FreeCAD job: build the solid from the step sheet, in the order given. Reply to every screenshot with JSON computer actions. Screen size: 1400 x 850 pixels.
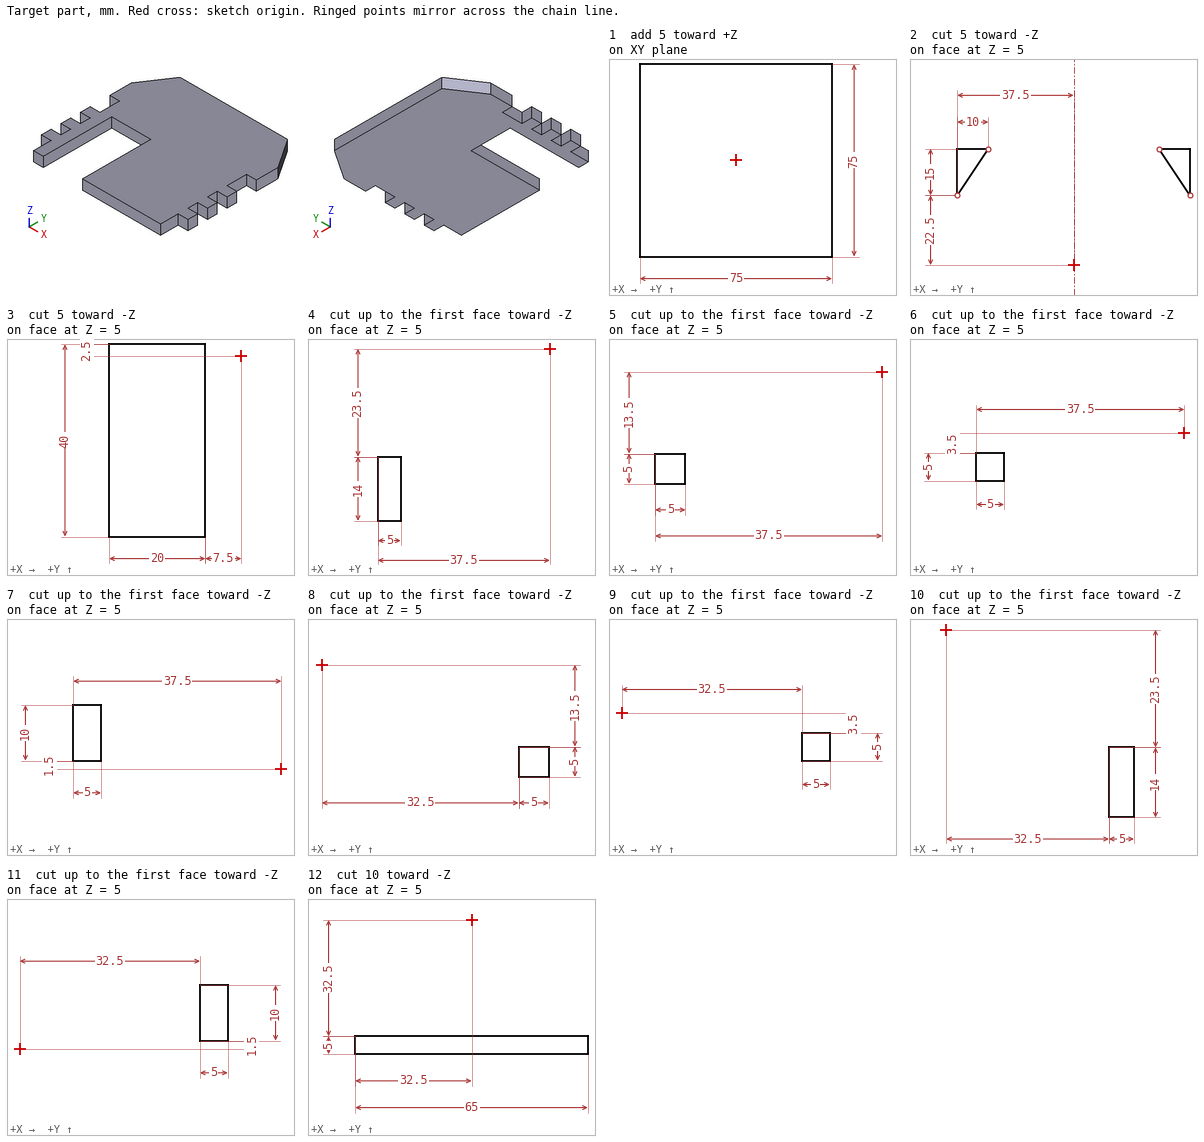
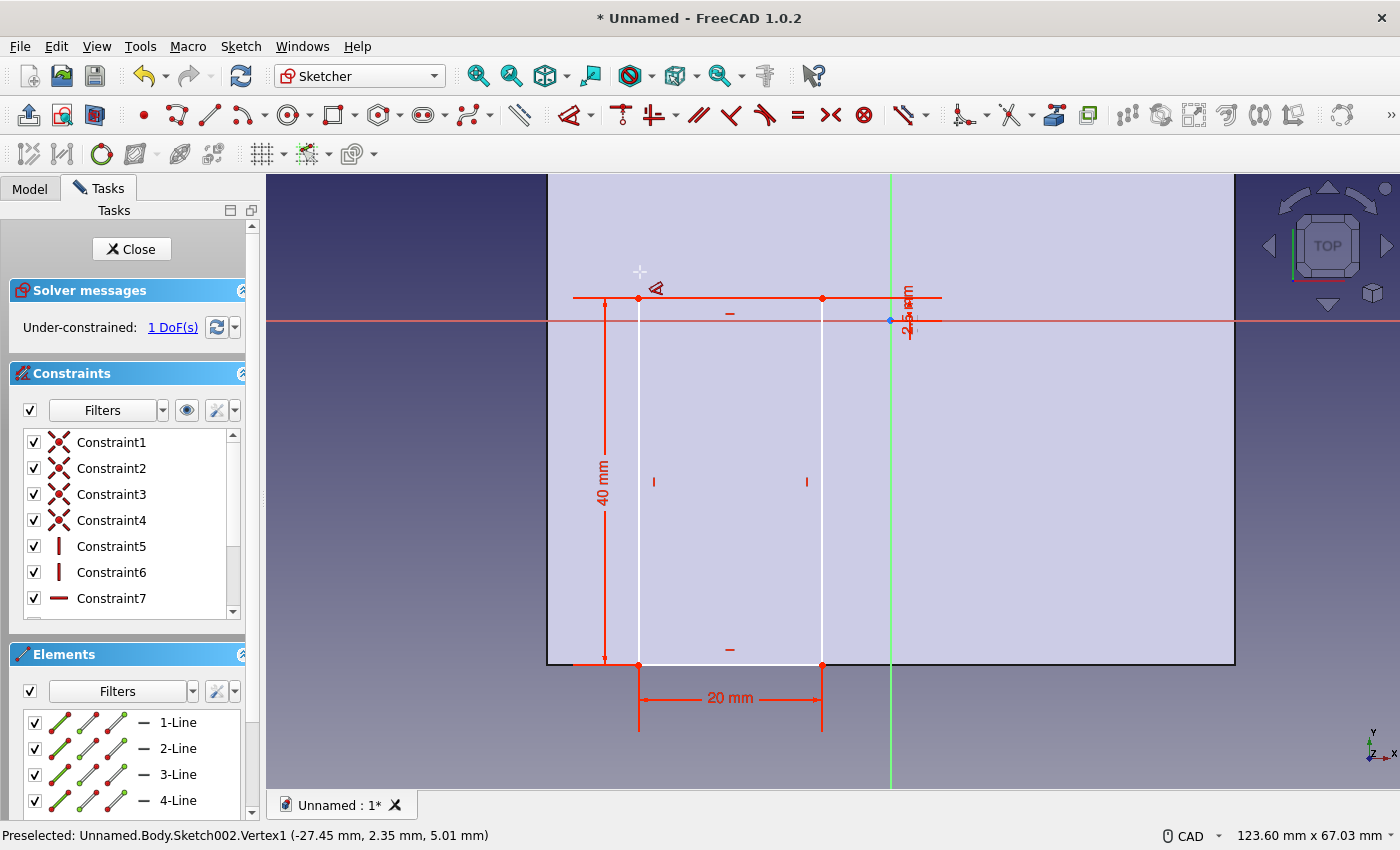
{"action": "left_click", "coordinate": [822, 665]}
{"action": "left_click", "coordinate": [857, 699]}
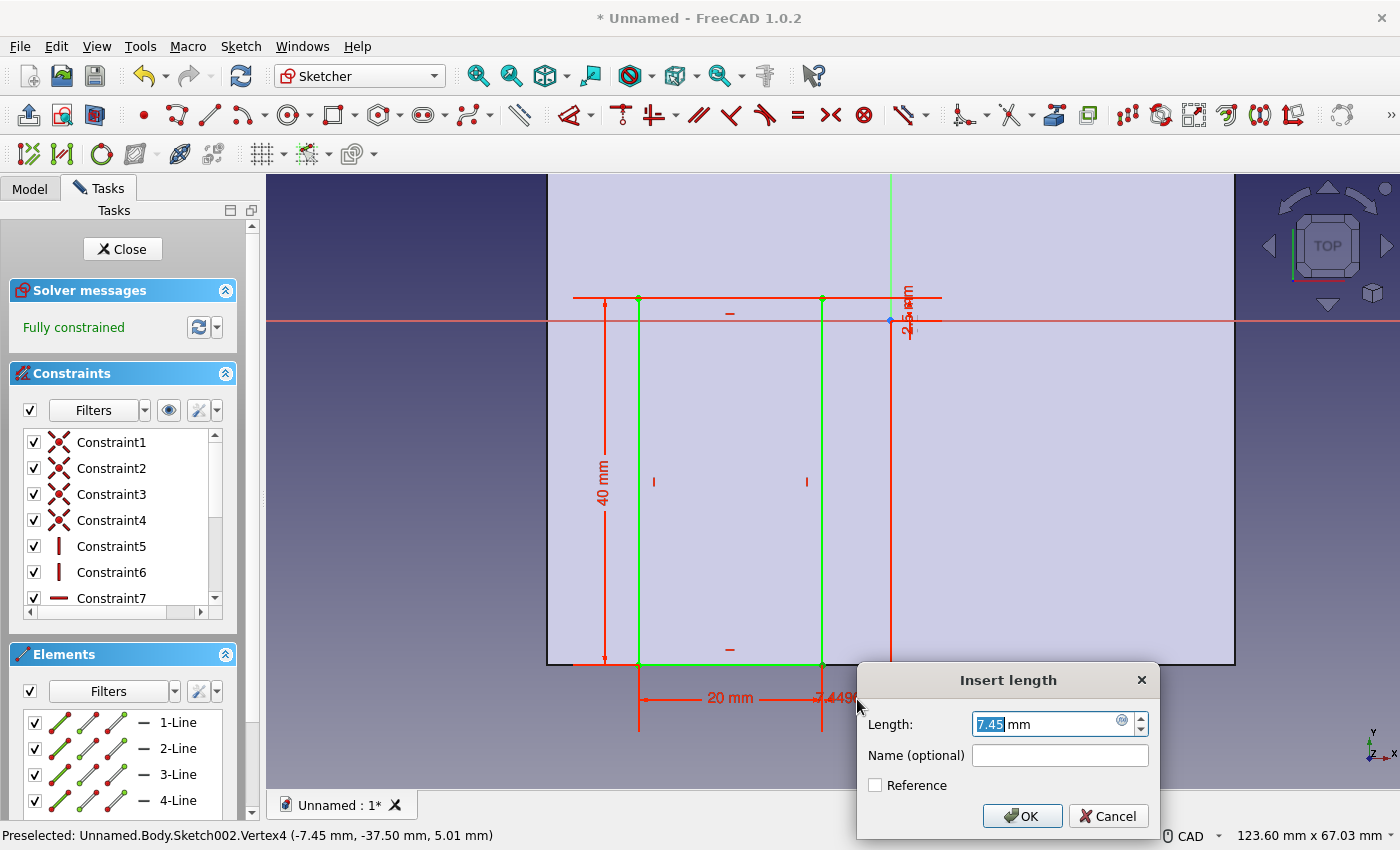
{"action": "type", "text": "7.5"}
{"action": "key", "text": "Return"}
{"action": "key", "text": "Escape"}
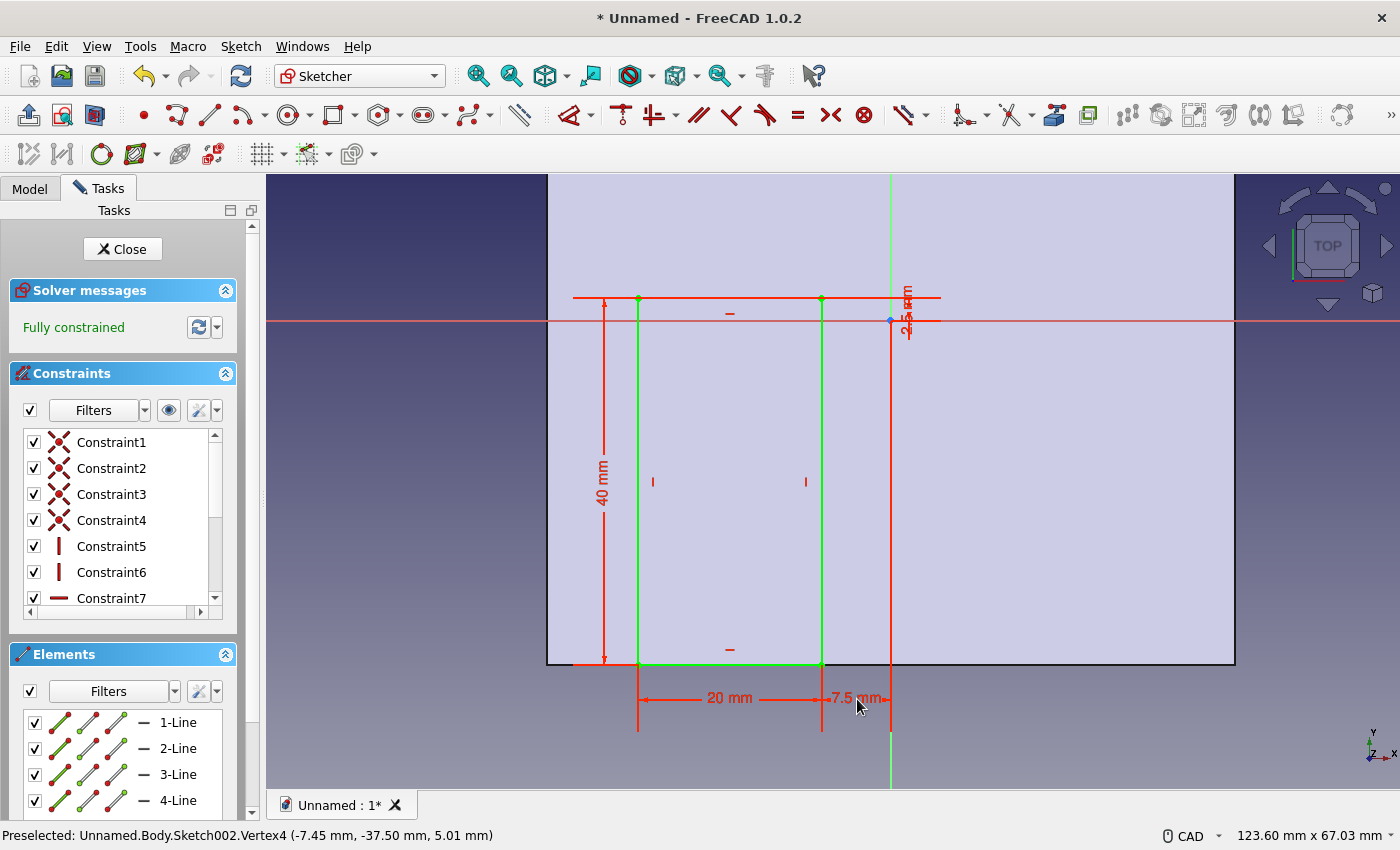
{"action": "left_click", "coordinate": [123, 249]}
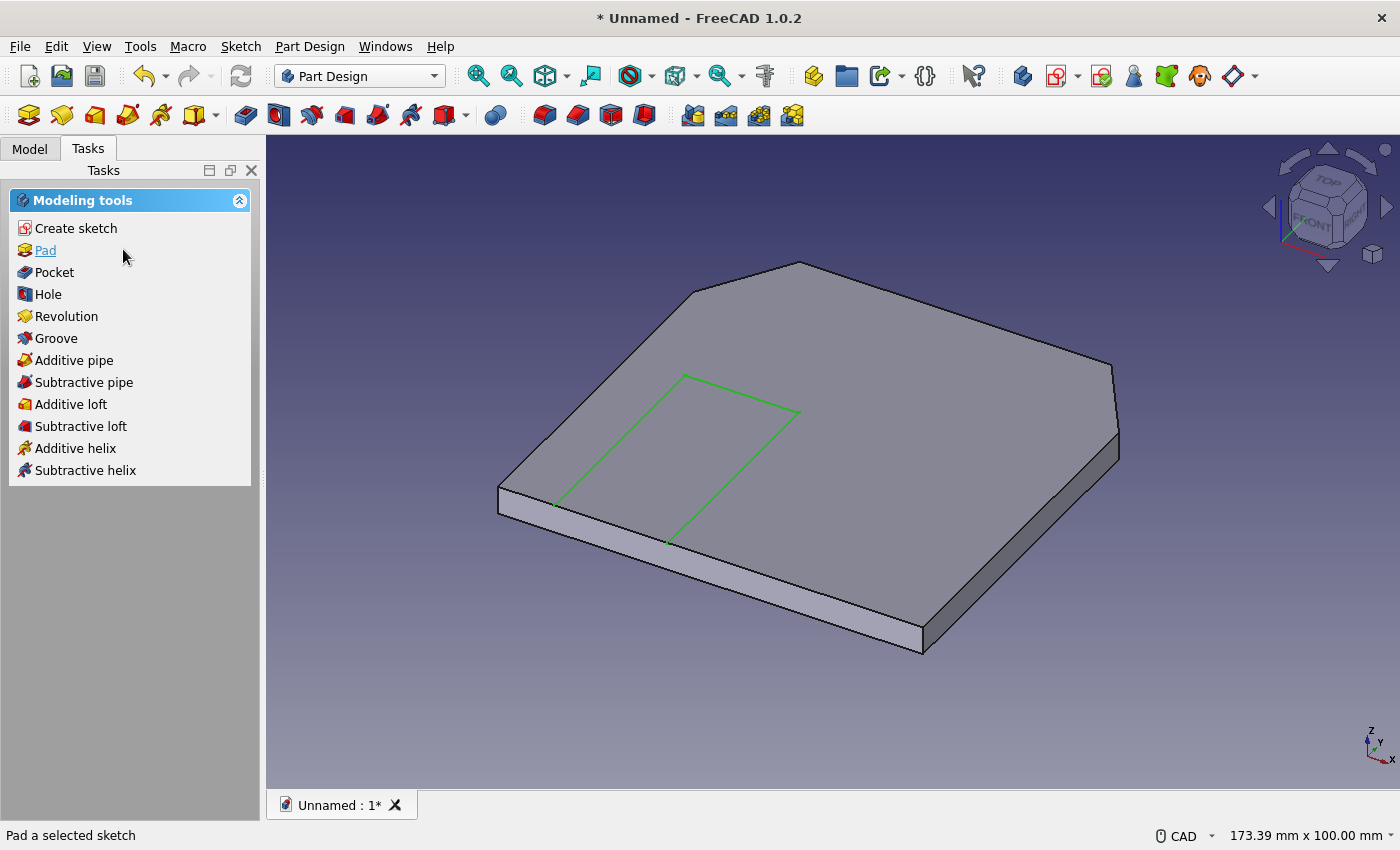
{"action": "left_click", "coordinate": [246, 116]}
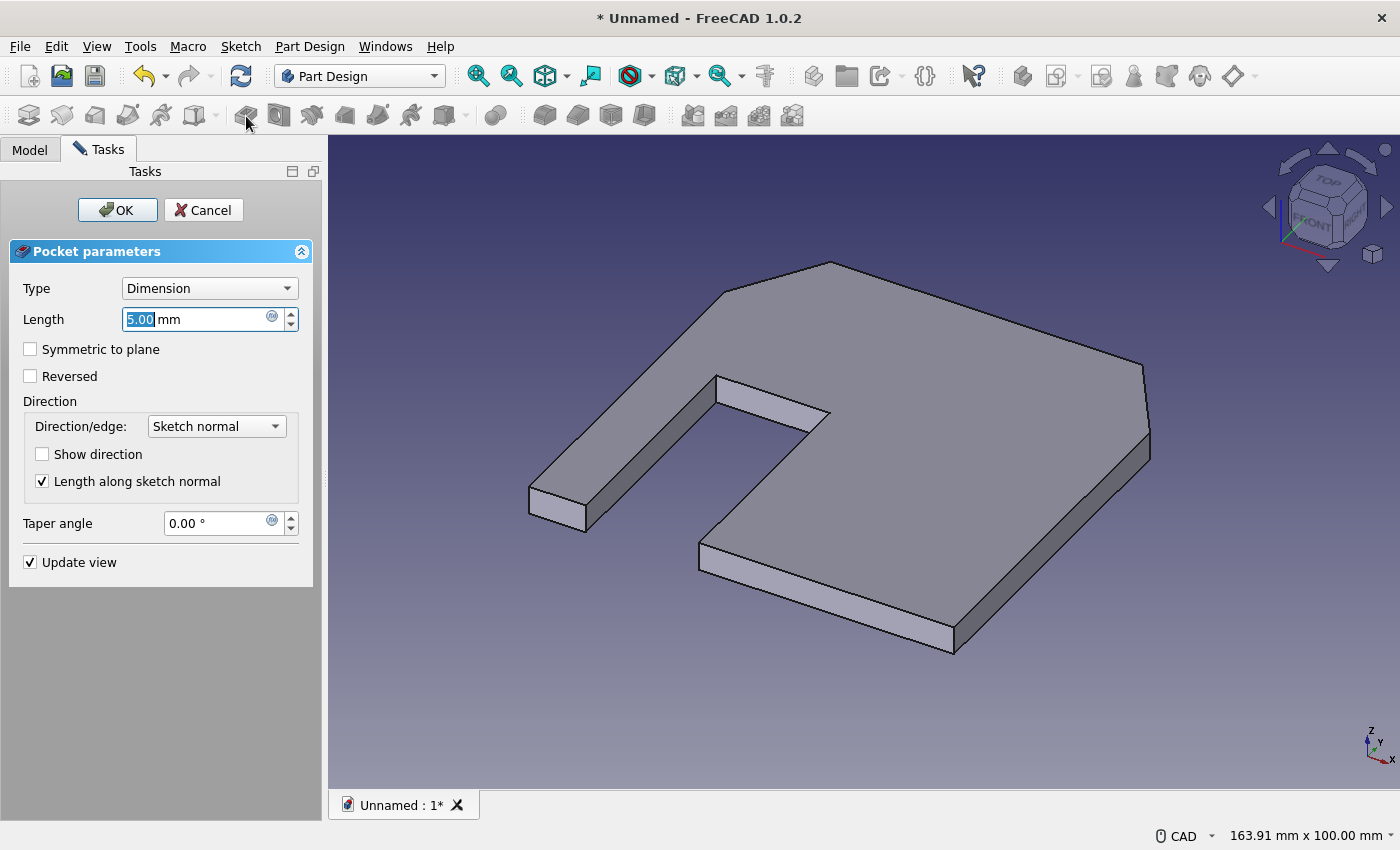
{"action": "type", "text": "5"}
{"action": "key", "text": "Tab"}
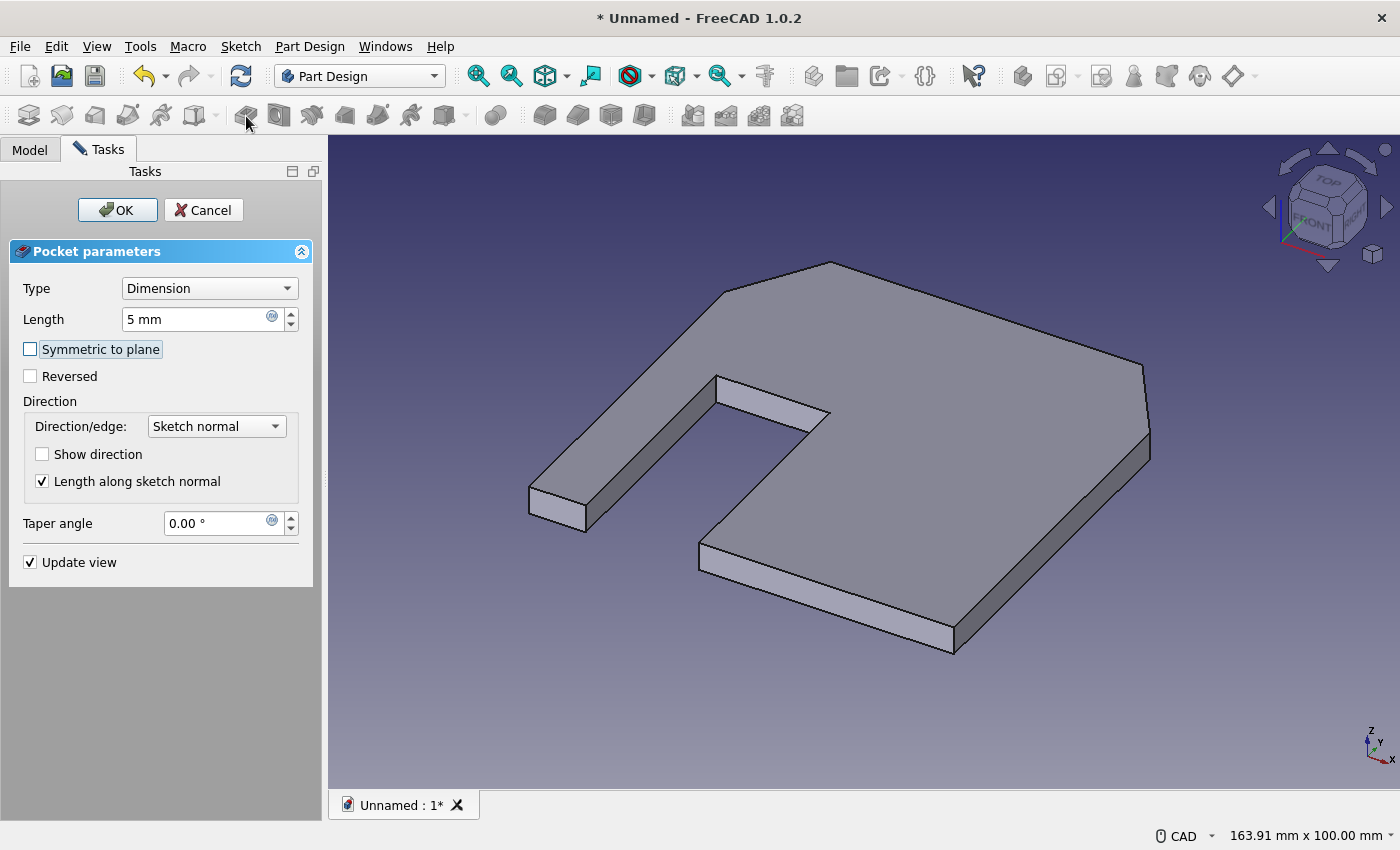
{"action": "left_click", "coordinate": [118, 210]}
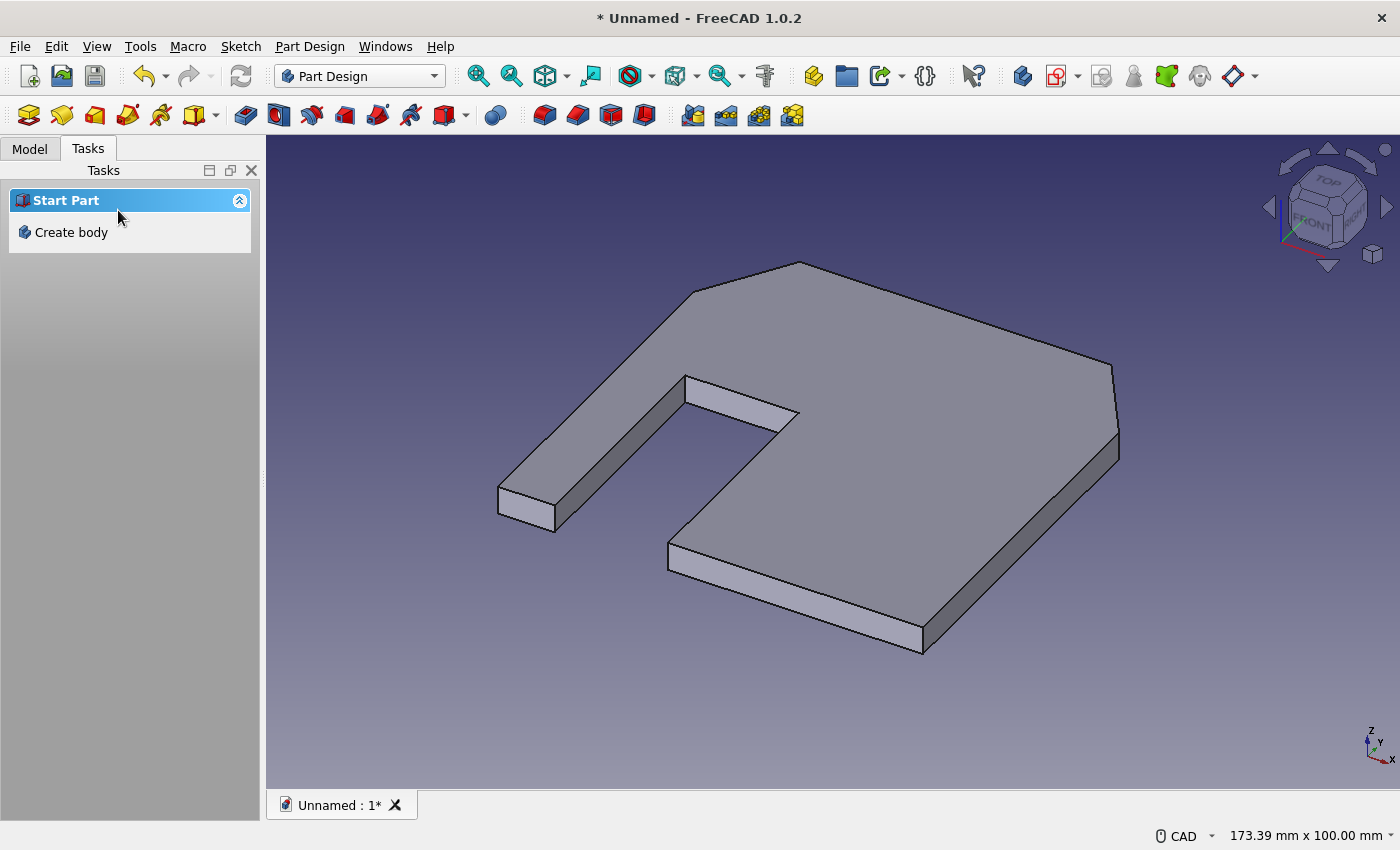
{"action": "left_click", "coordinate": [929, 420]}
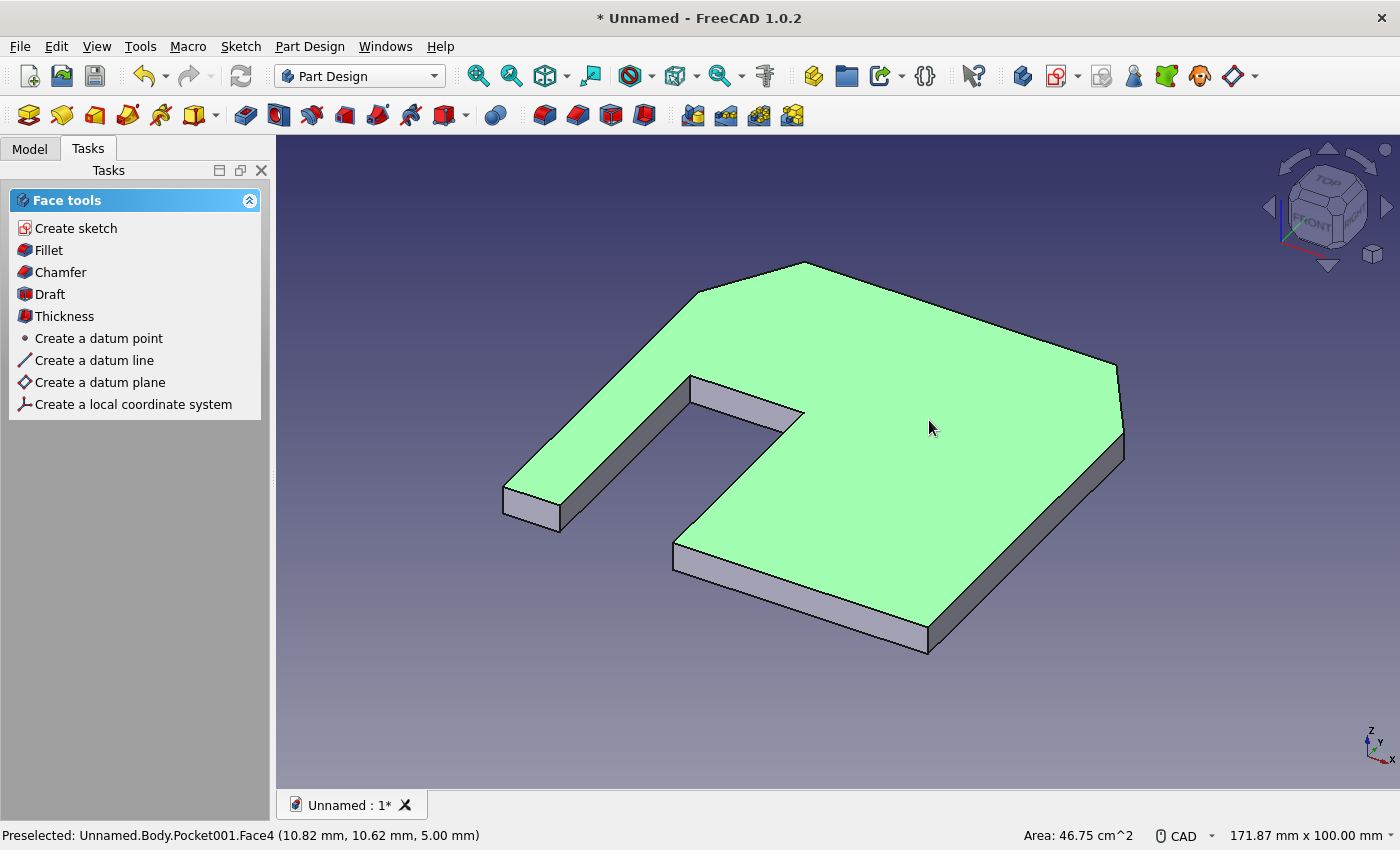
{"action": "left_click", "coordinate": [1056, 76]}